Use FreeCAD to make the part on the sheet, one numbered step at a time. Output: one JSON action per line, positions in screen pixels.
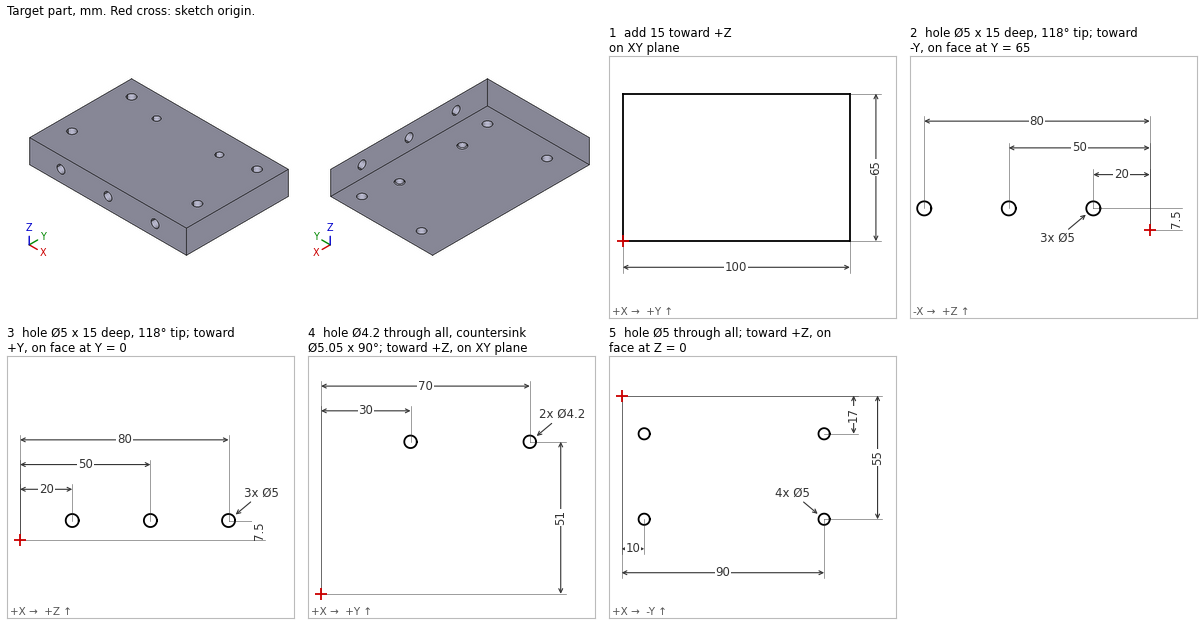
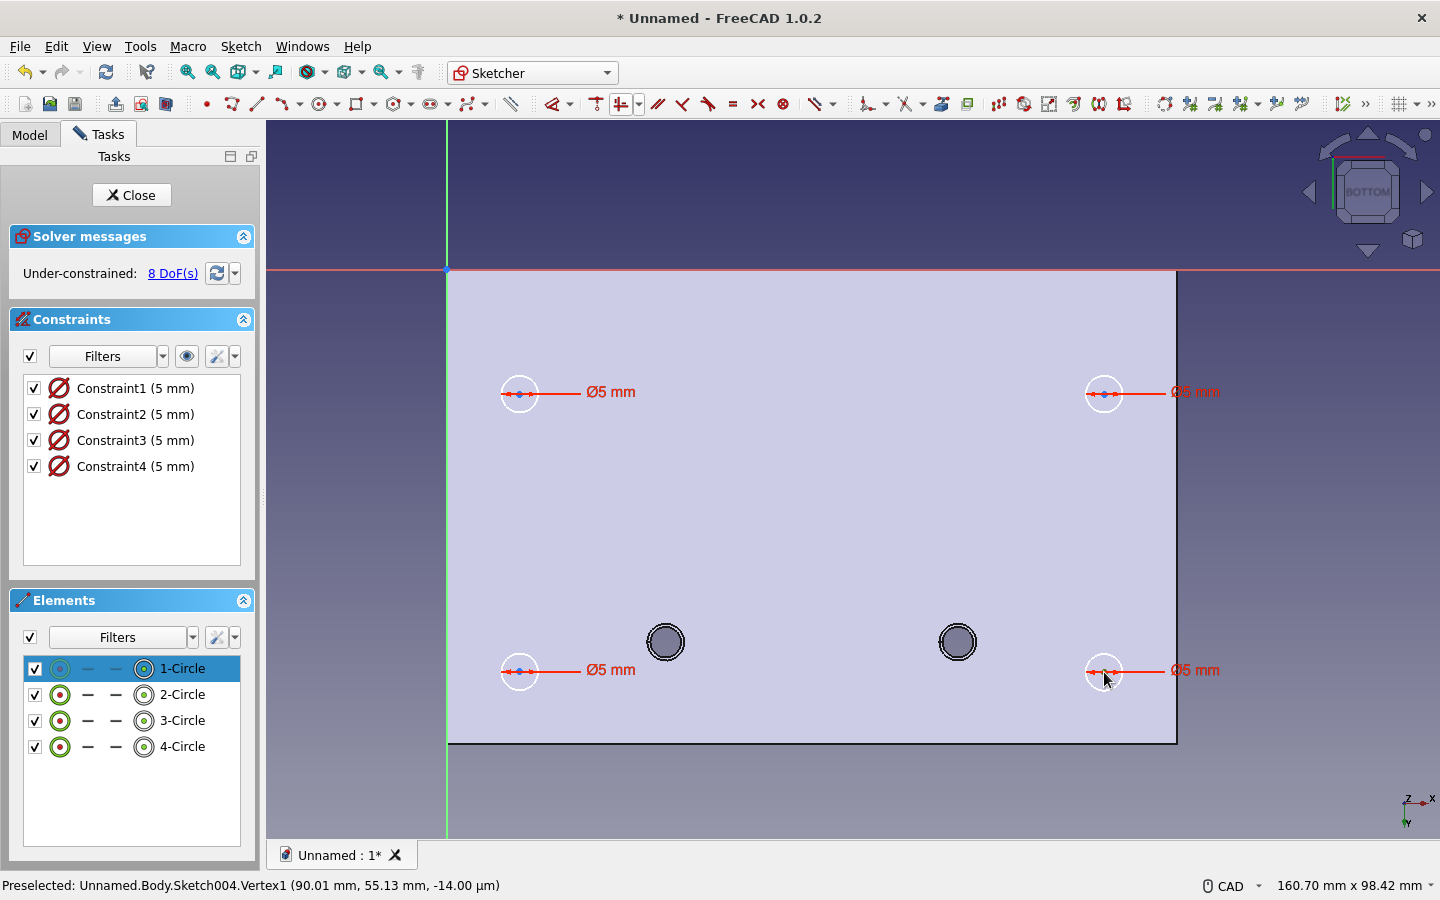
{"action": "left_click", "coordinate": [520, 672]}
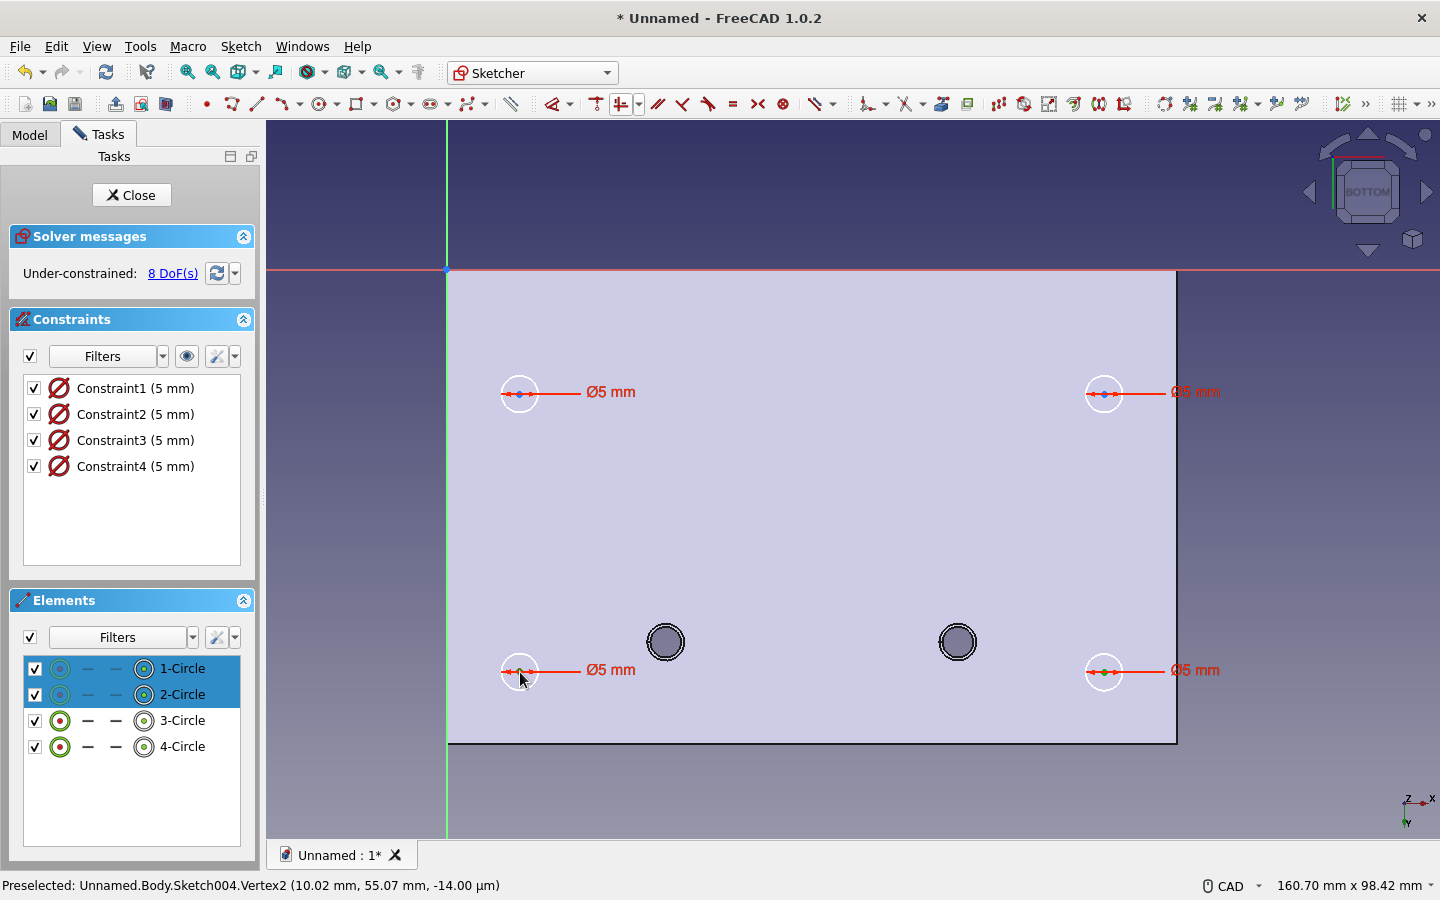
{"action": "key", "text": "h"}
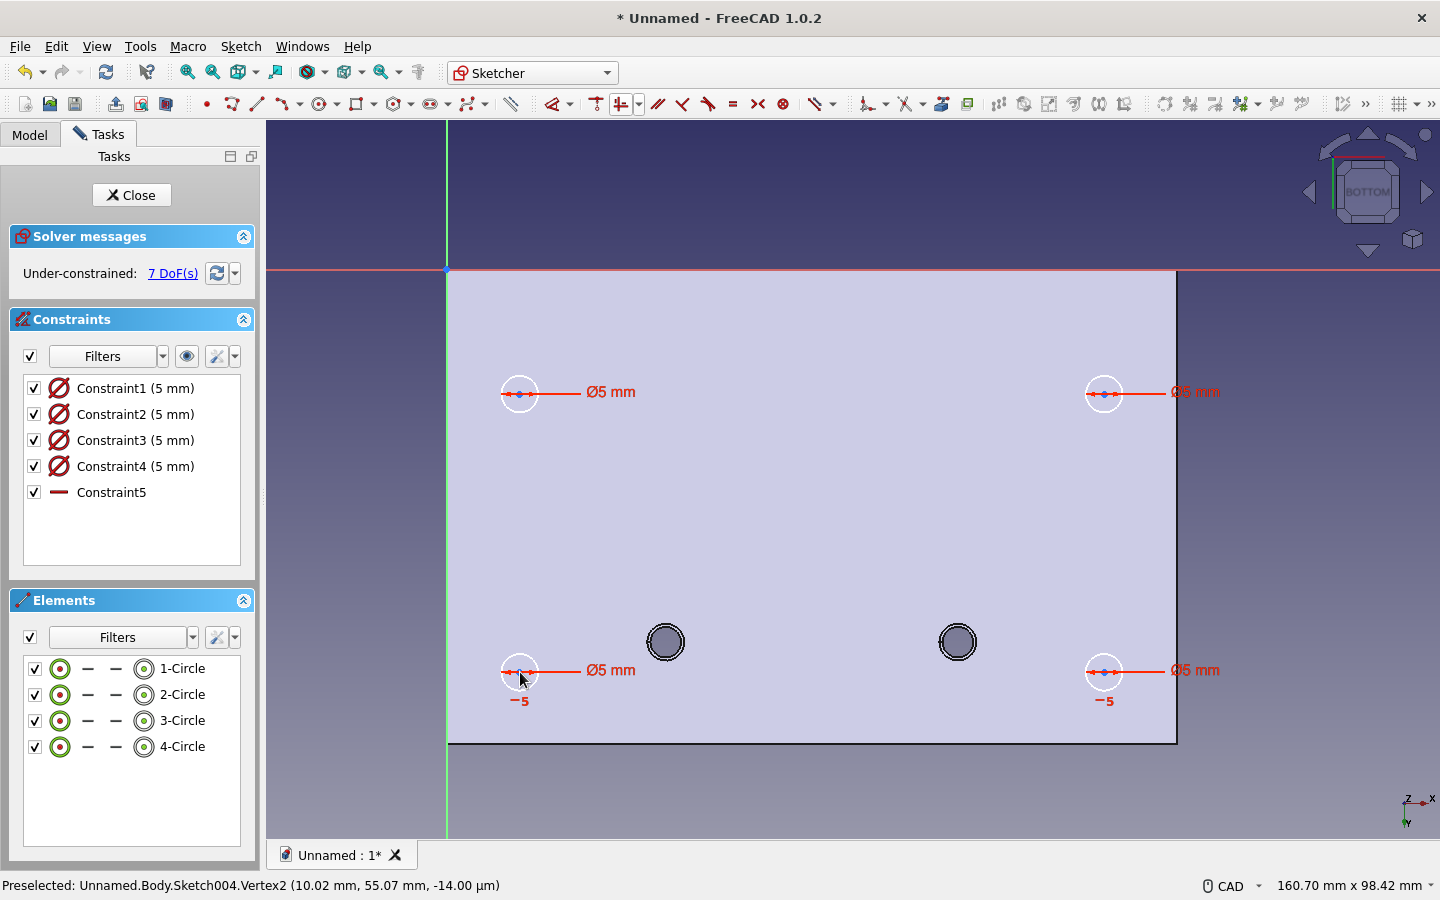
{"action": "left_click", "coordinate": [1104, 672]}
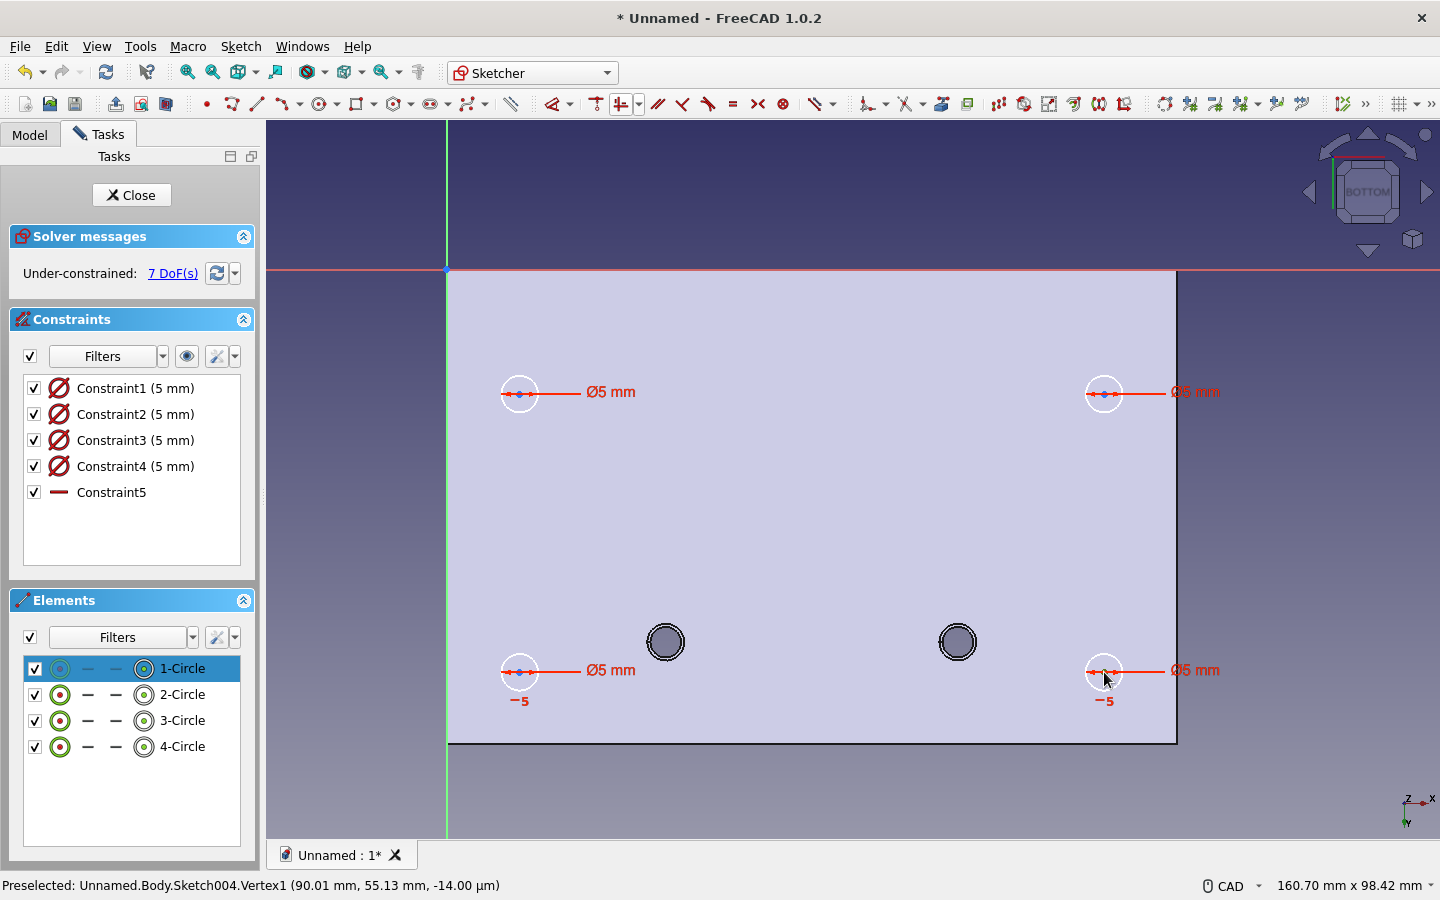
{"action": "left_click", "coordinate": [1104, 394]}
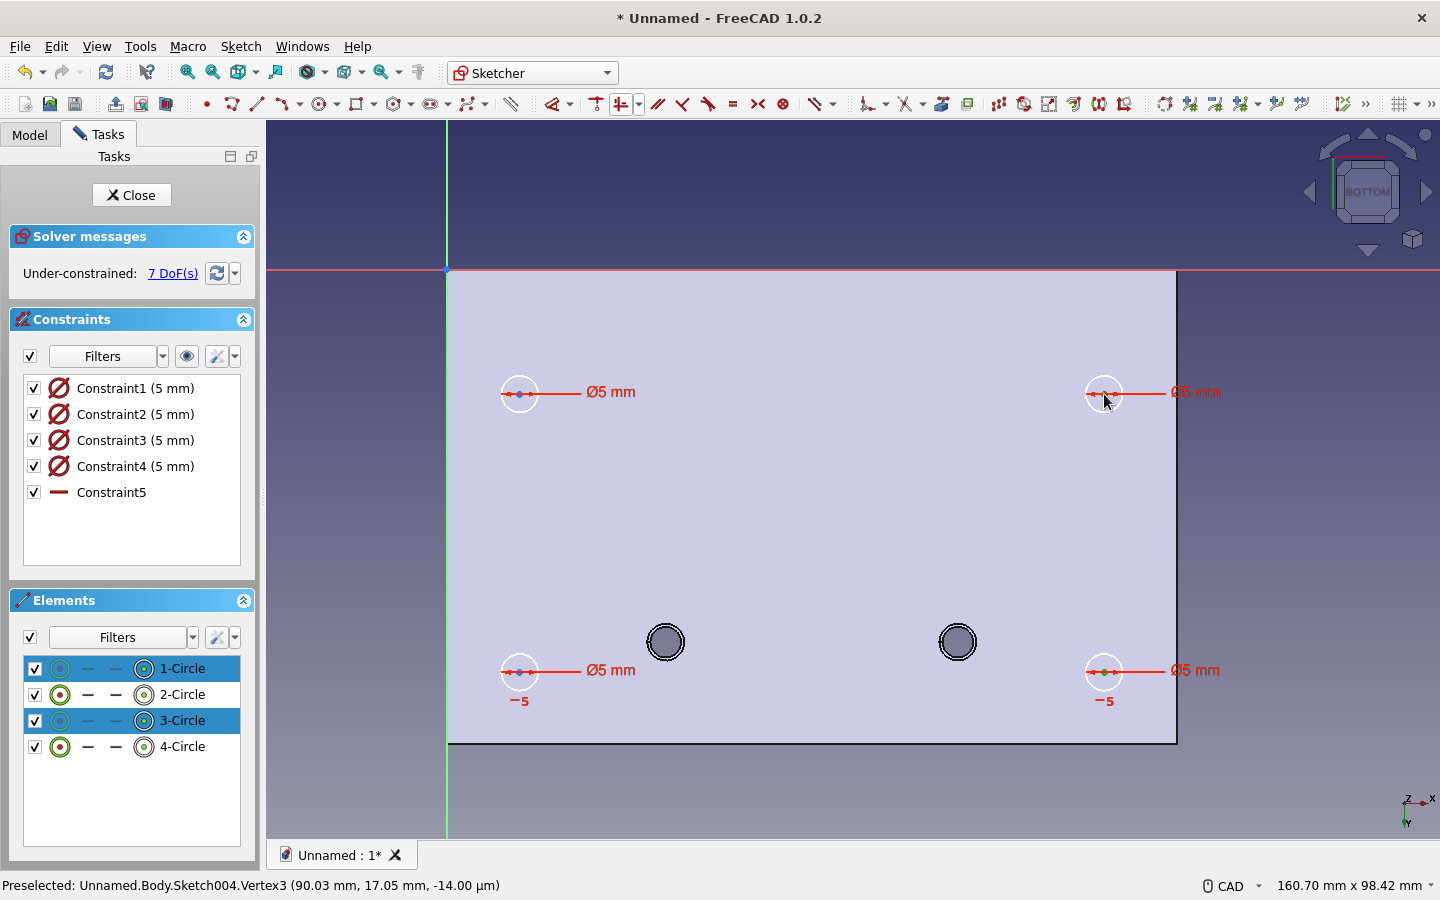
{"action": "key", "text": "v"}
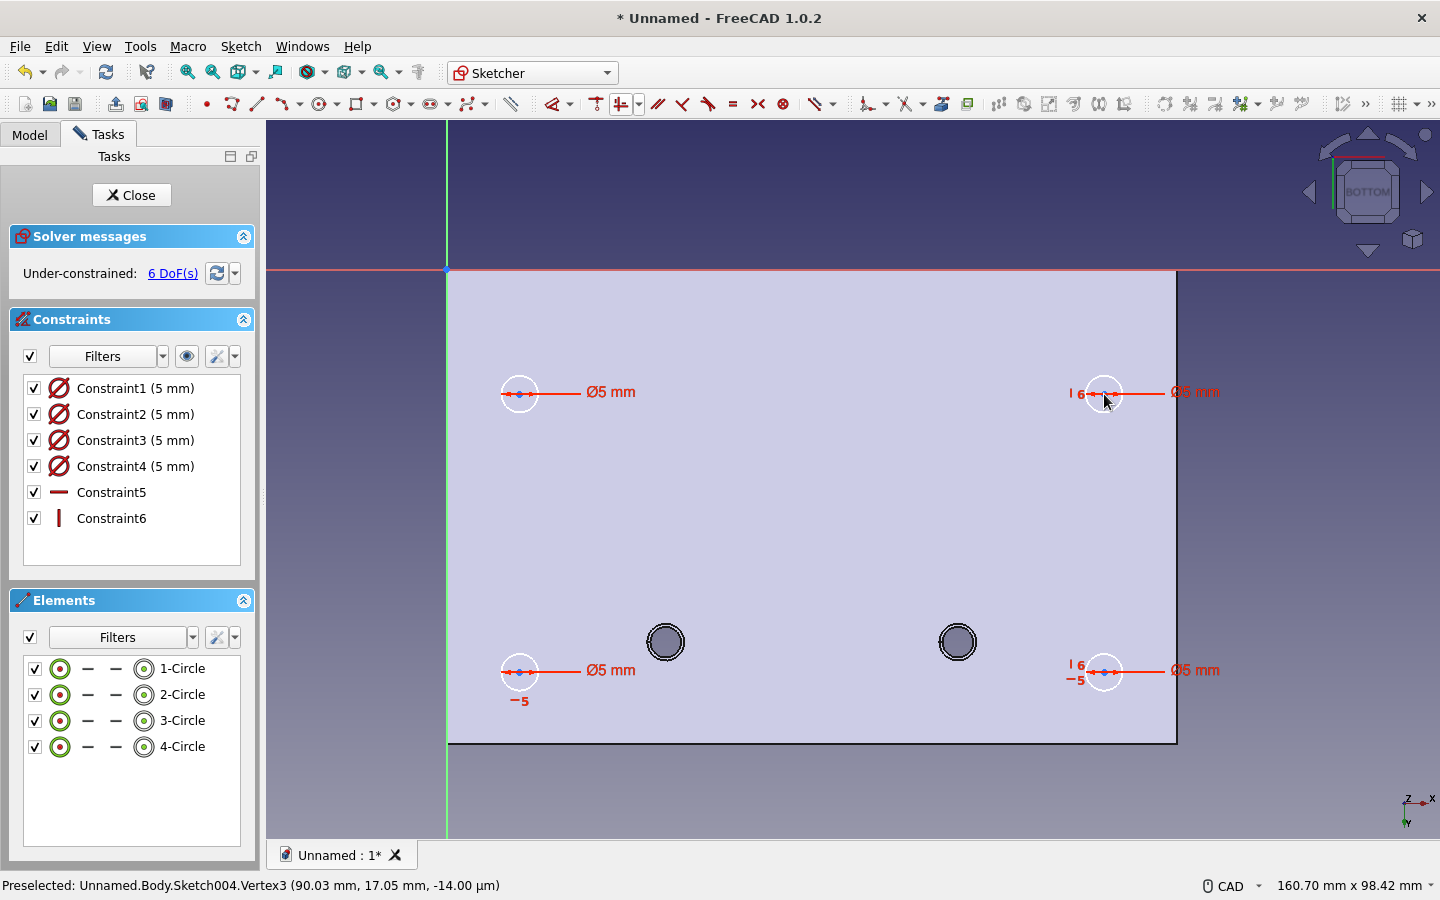
{"action": "left_click", "coordinate": [520, 672]}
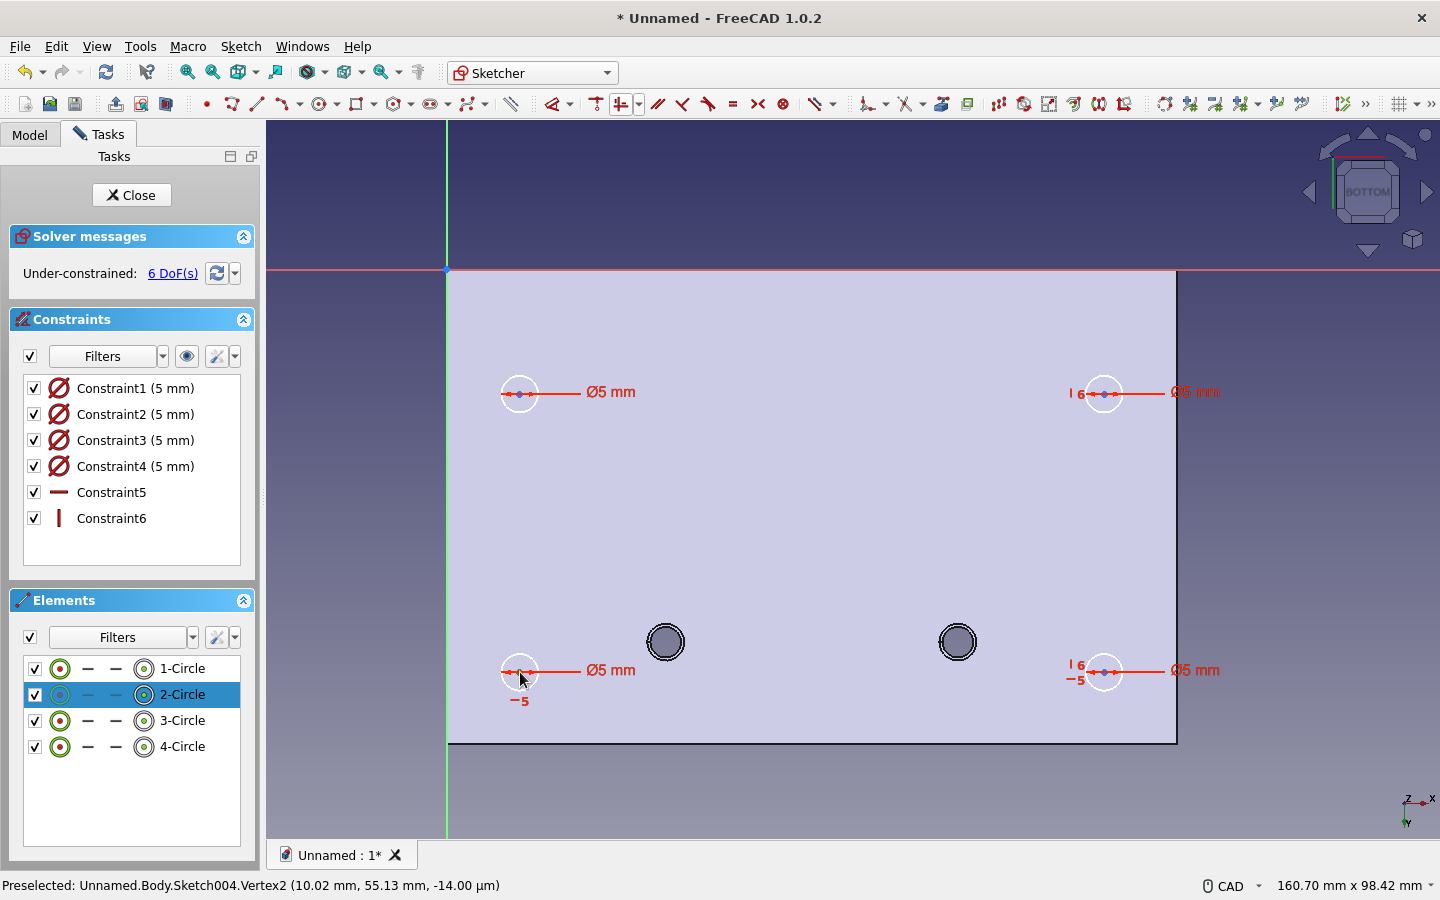
{"action": "left_click", "coordinate": [520, 394]}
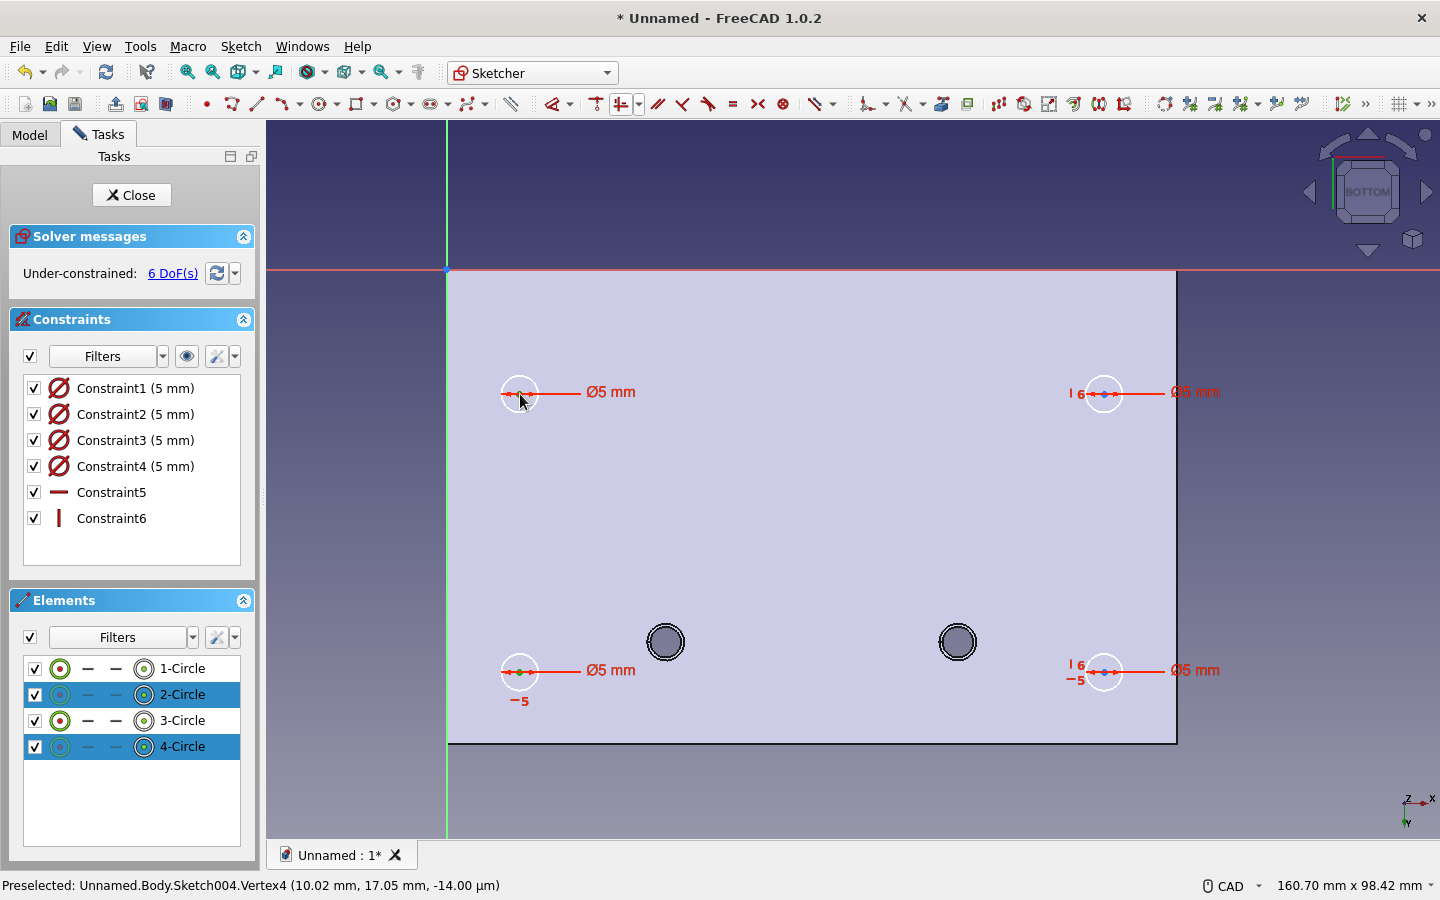
{"action": "left_click", "coordinate": [638, 104]}